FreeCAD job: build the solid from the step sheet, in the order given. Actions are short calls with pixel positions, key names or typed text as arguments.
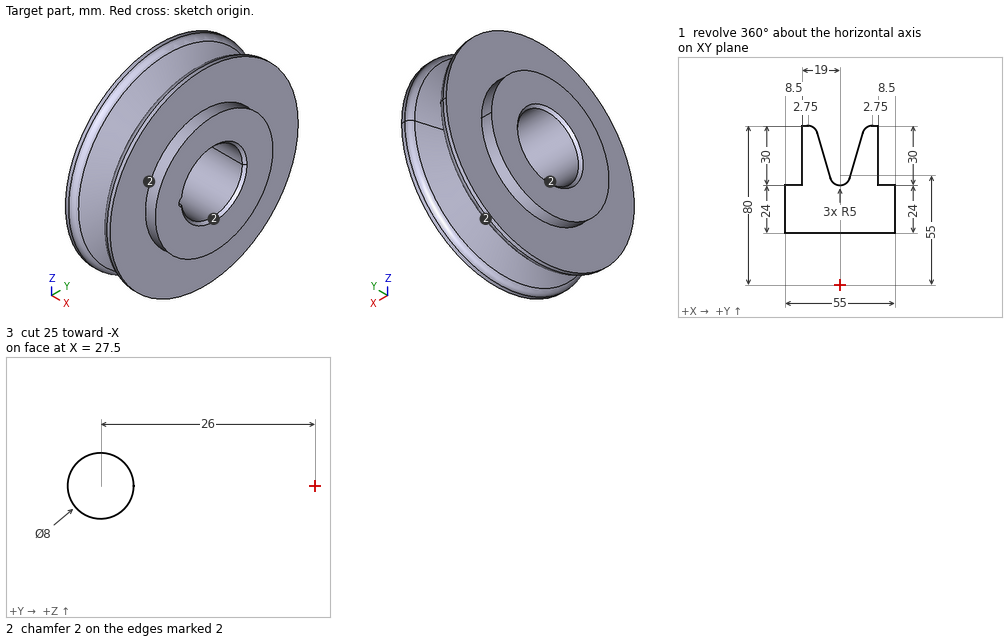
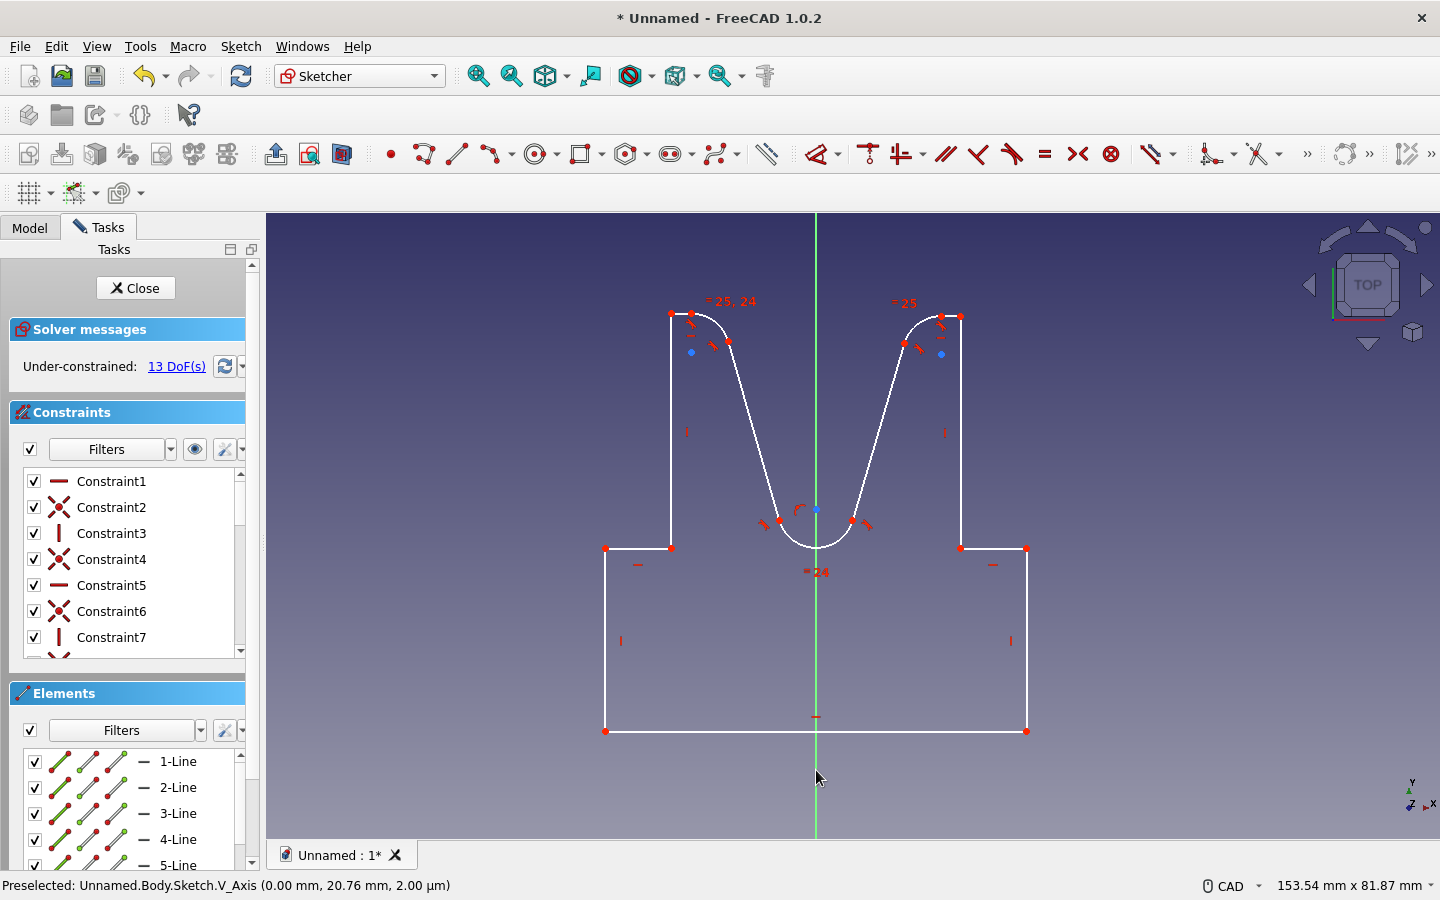
click(797, 543)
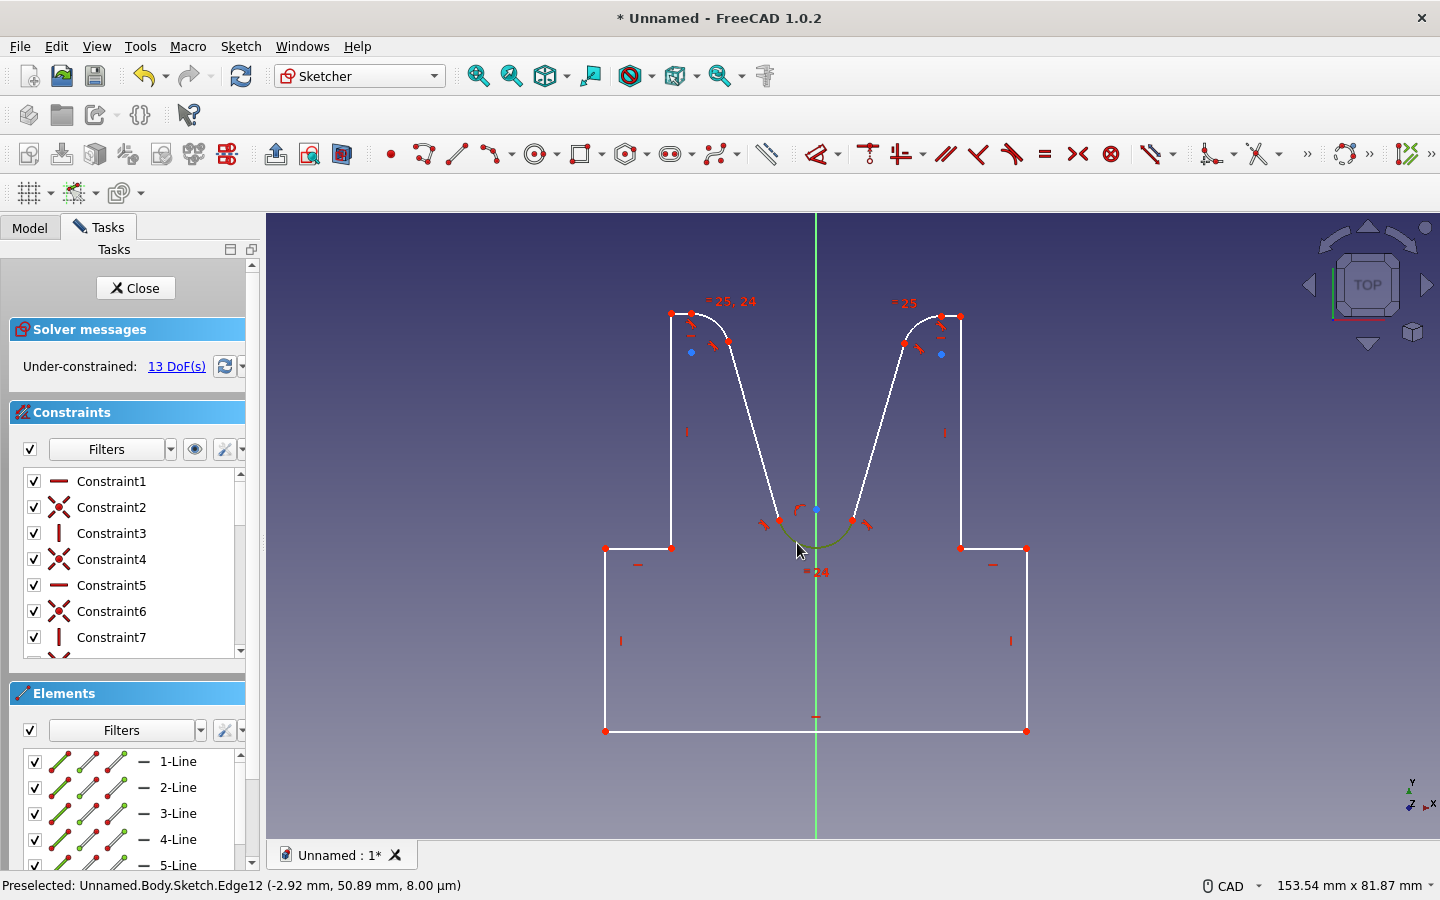
click(838, 154)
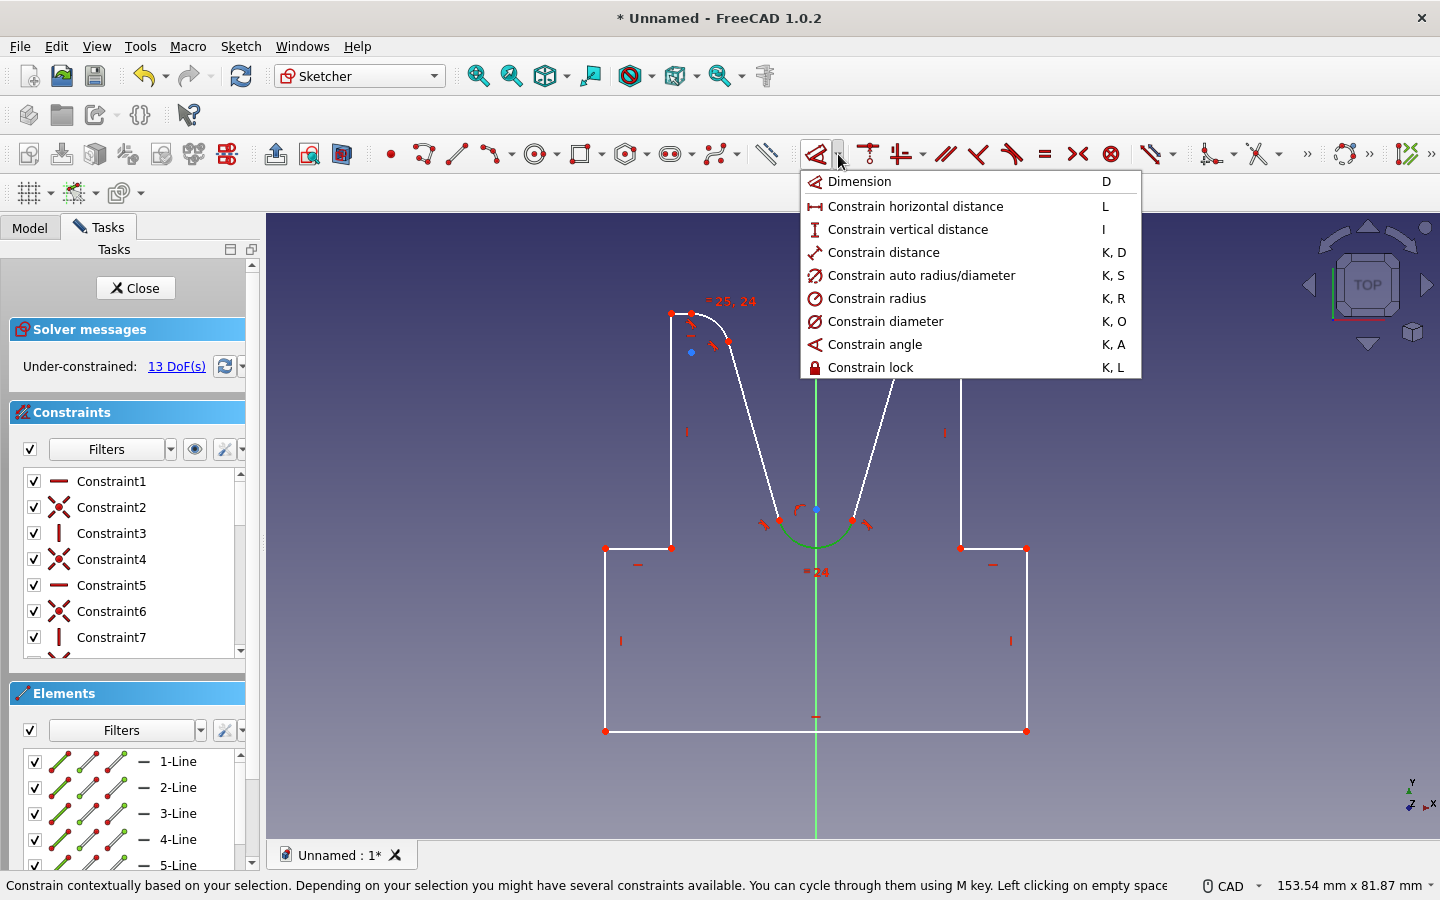
click(971, 298)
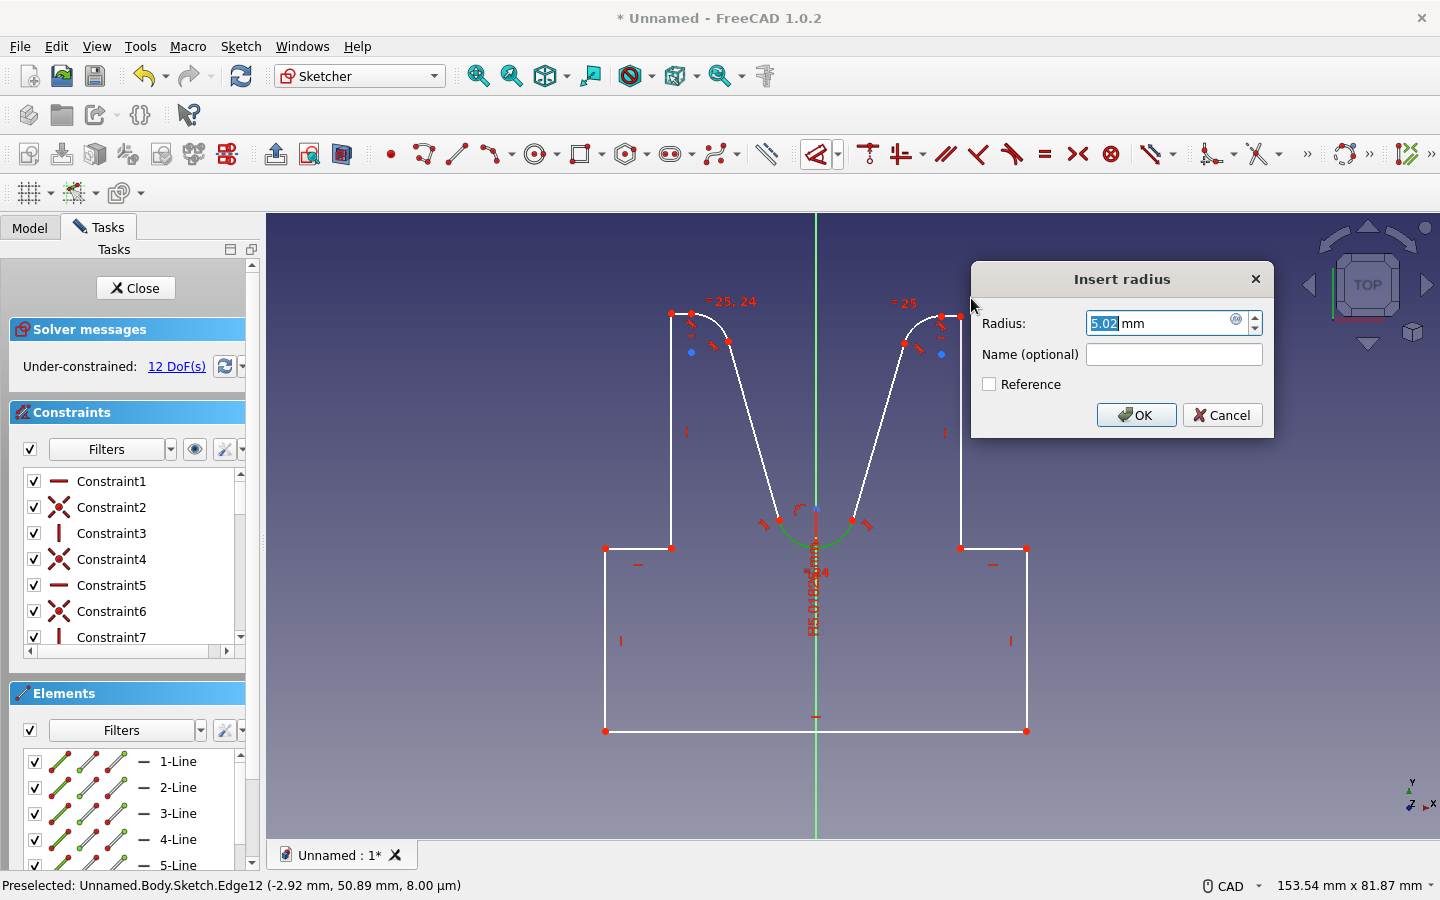
text(5)
key(Return)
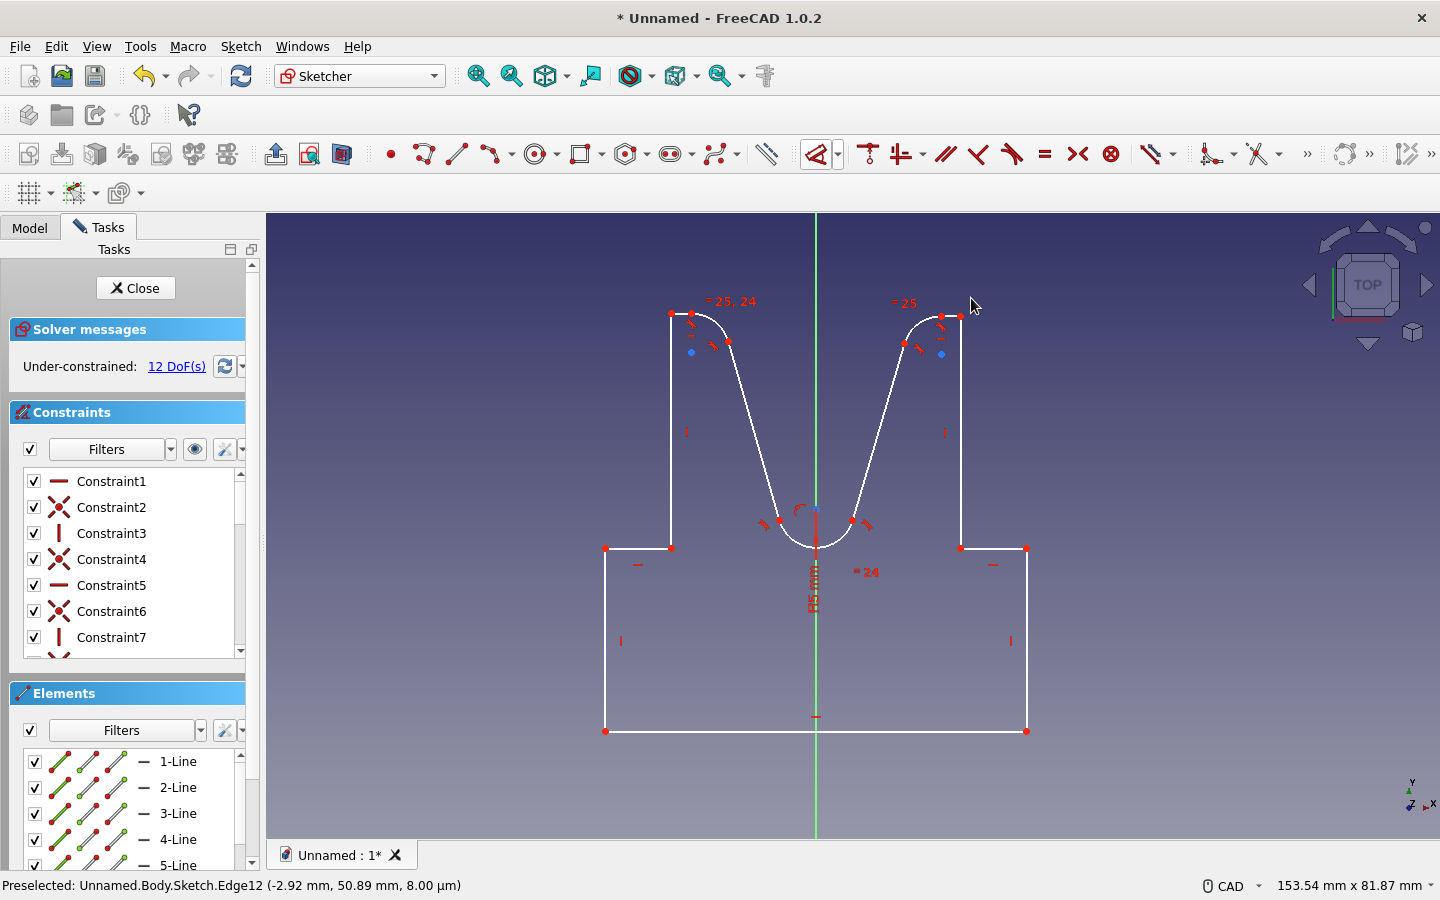
click(671, 384)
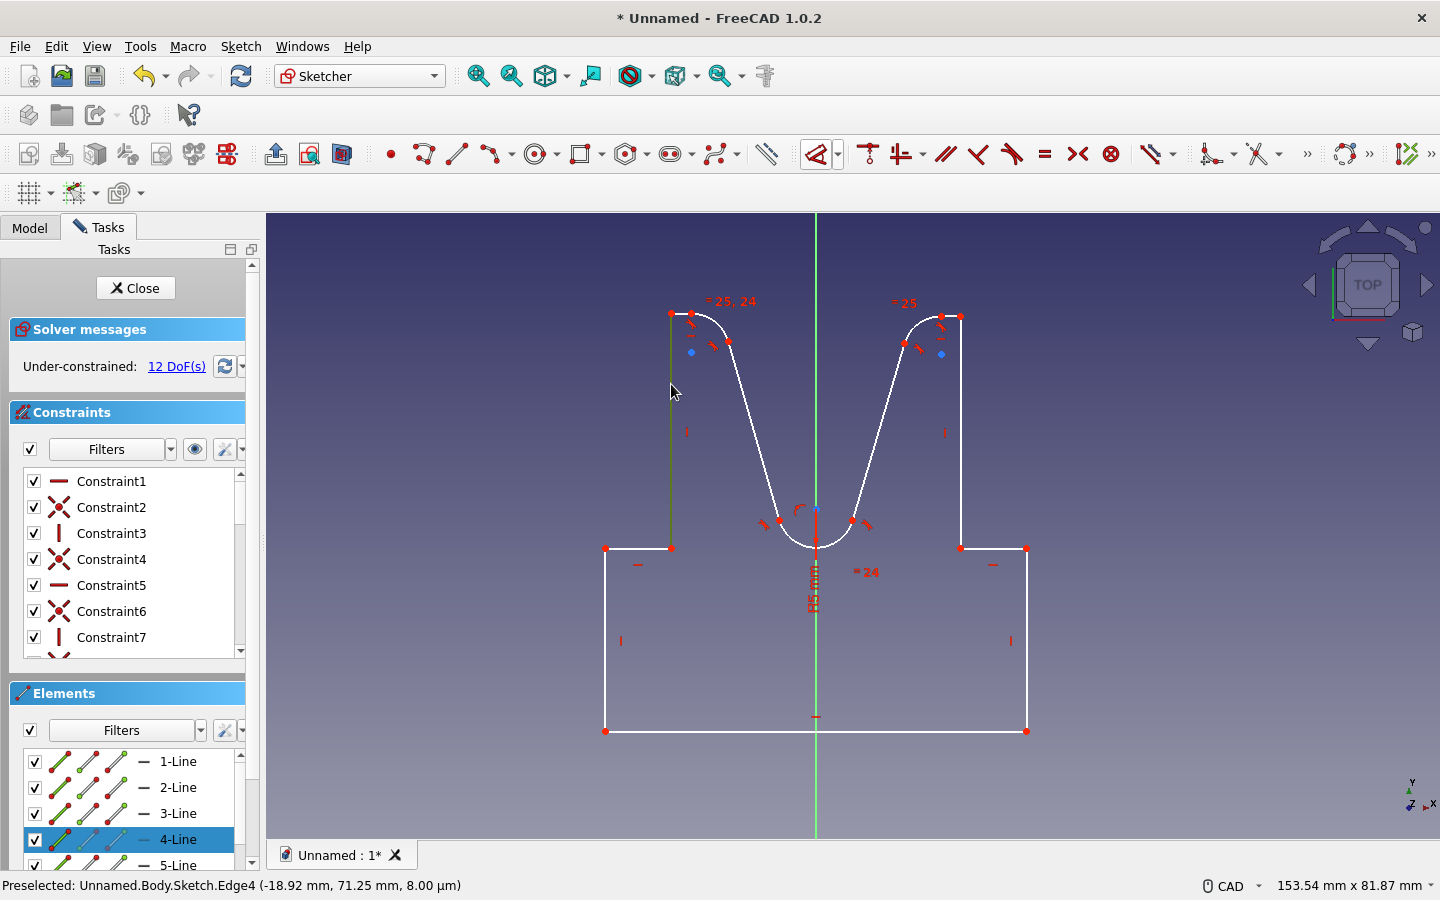
key(i)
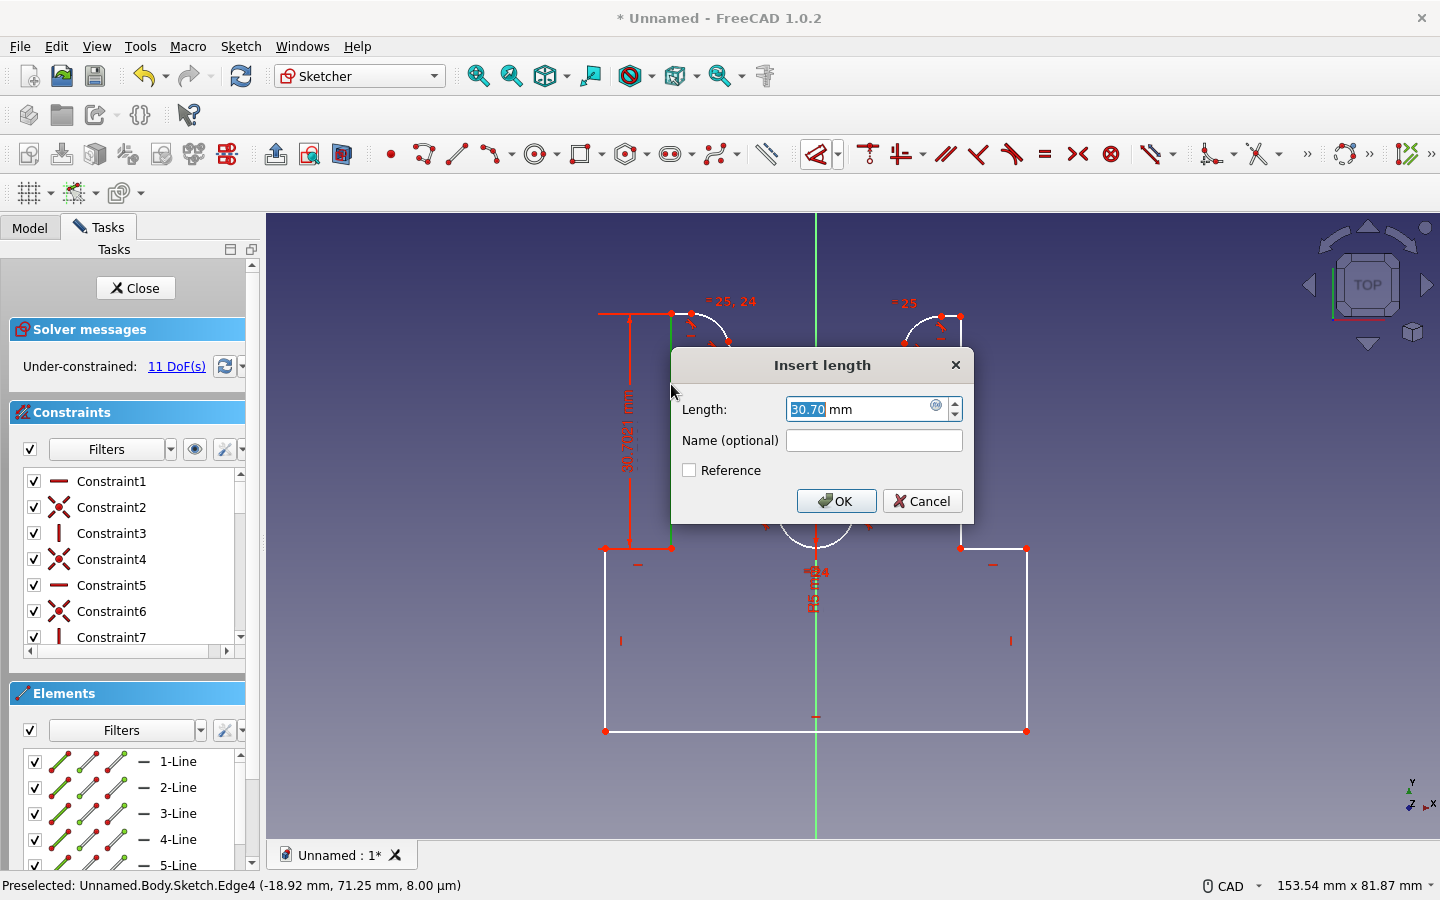
text(30)
key(Return)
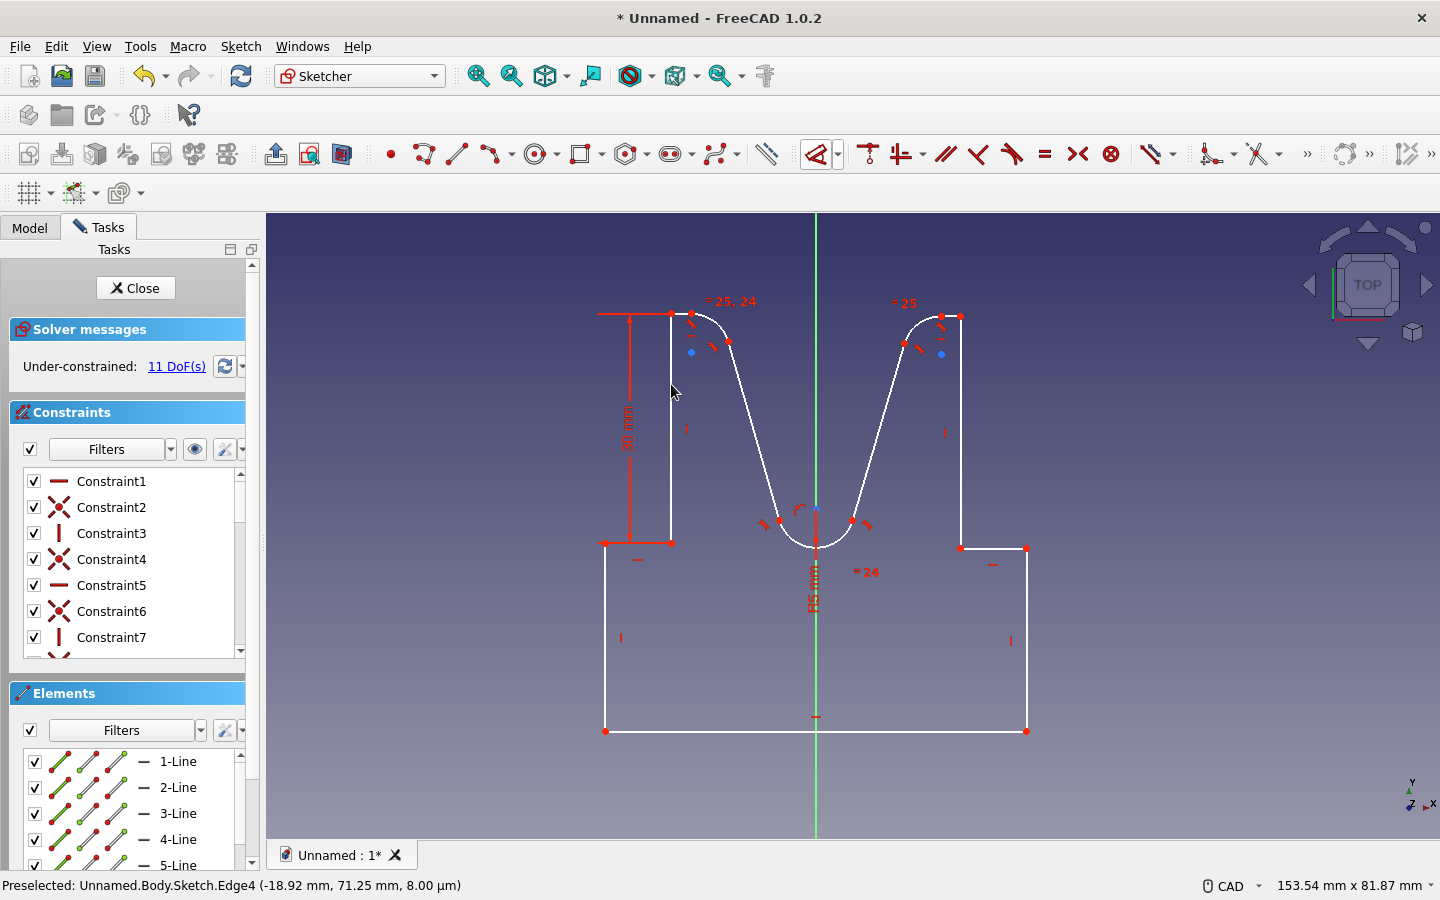
click(605, 600)